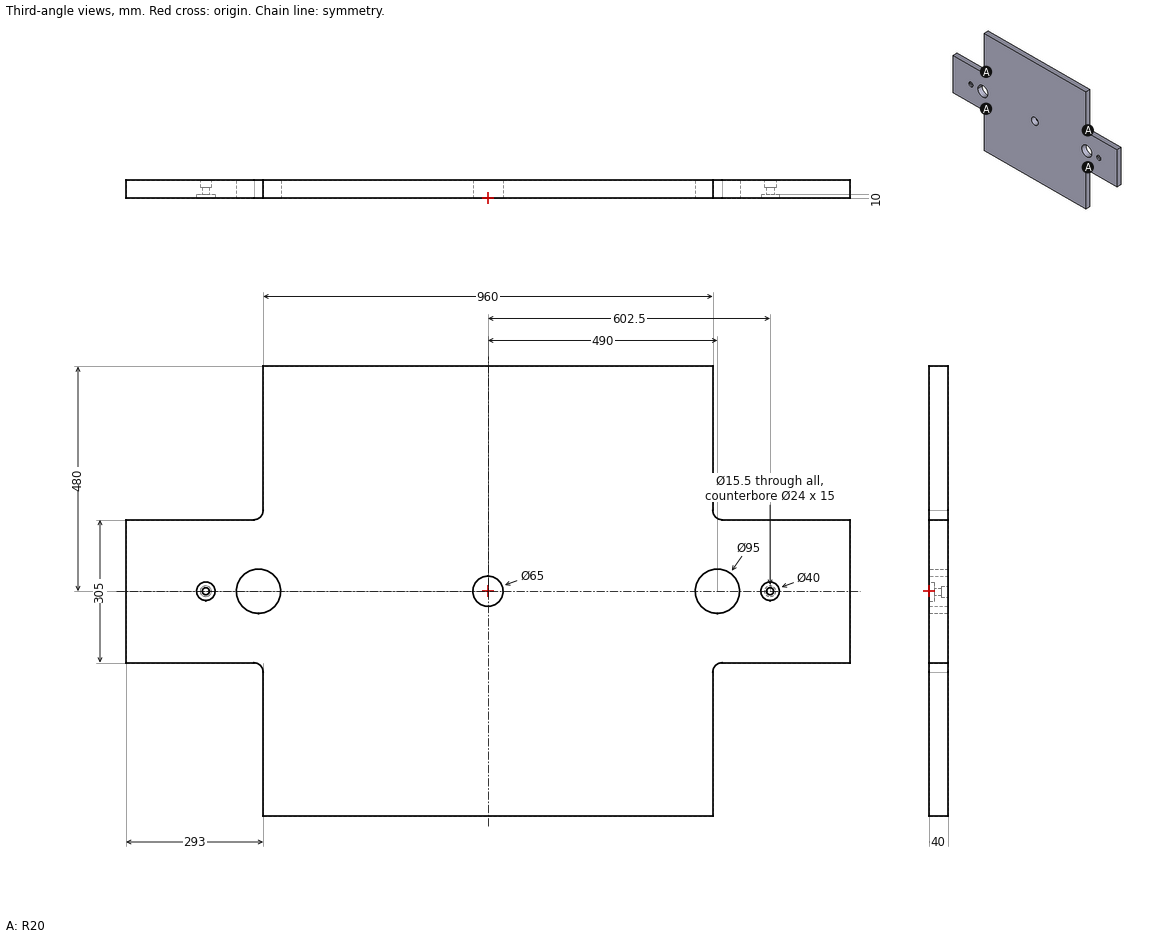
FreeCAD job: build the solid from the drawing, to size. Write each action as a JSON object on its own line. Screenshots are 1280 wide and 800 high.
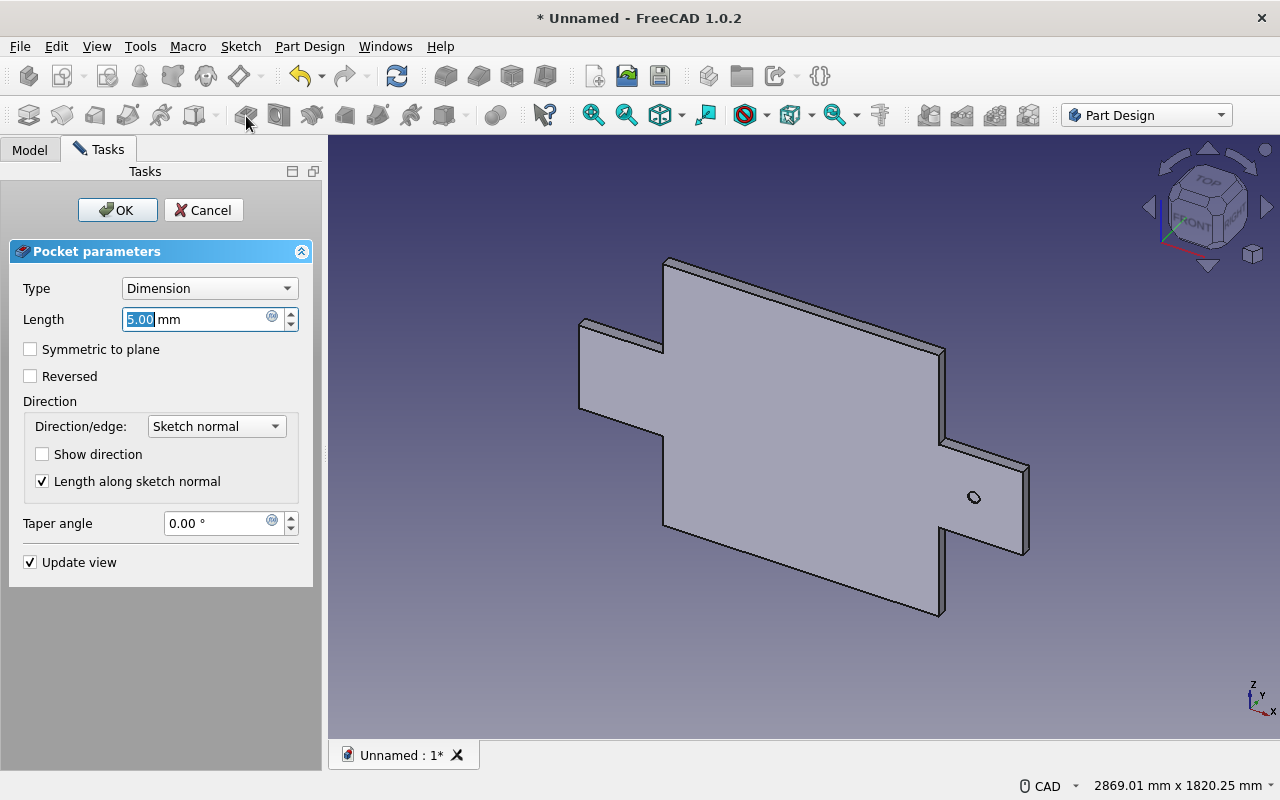
{"action": "type", "text": "10"}
{"action": "key", "text": "Tab"}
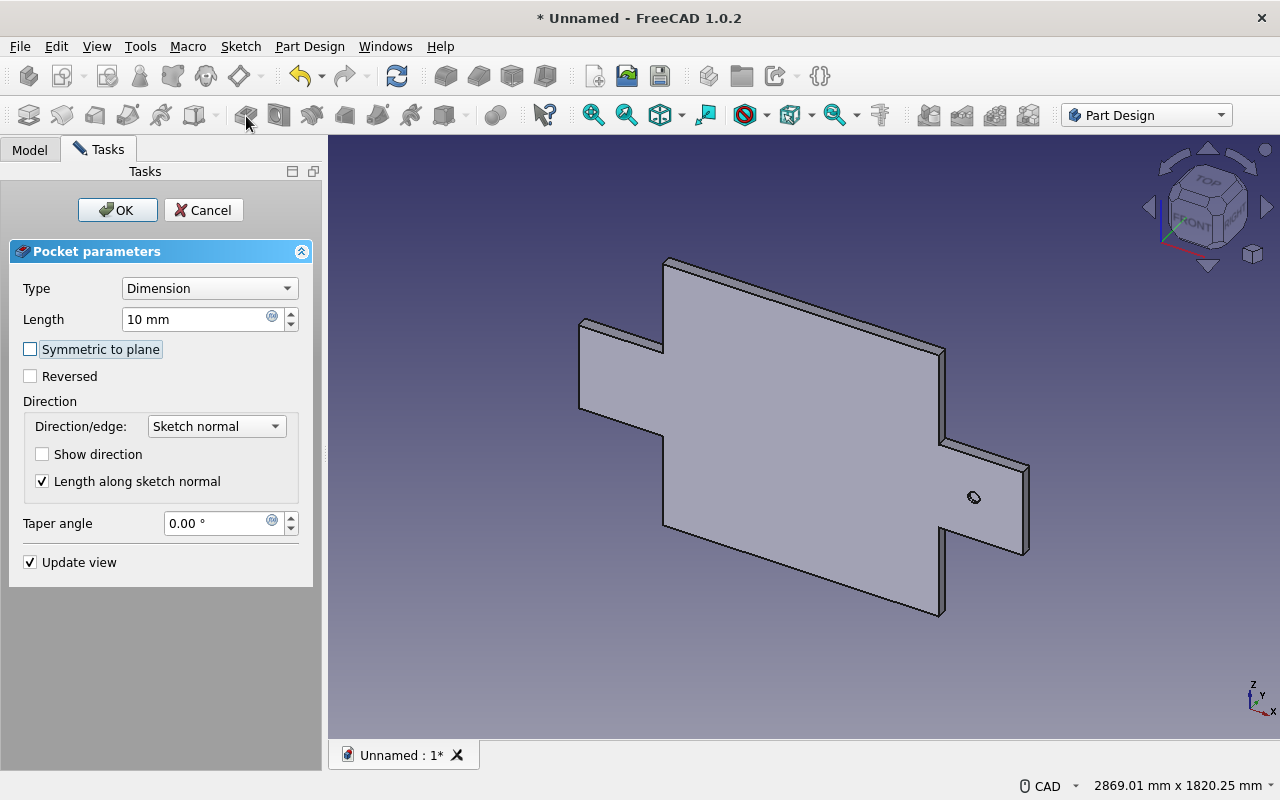
{"action": "left_click", "coordinate": [118, 210]}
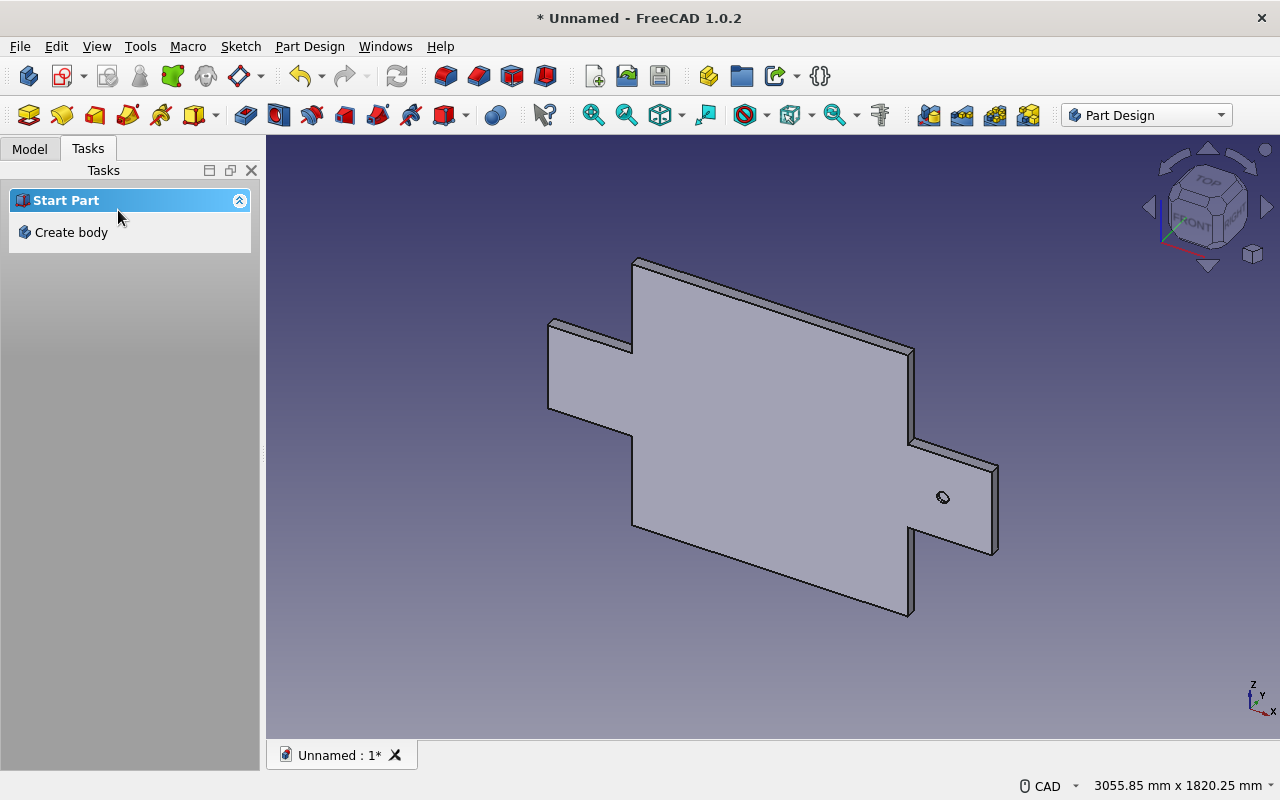
{"action": "key", "text": "4"}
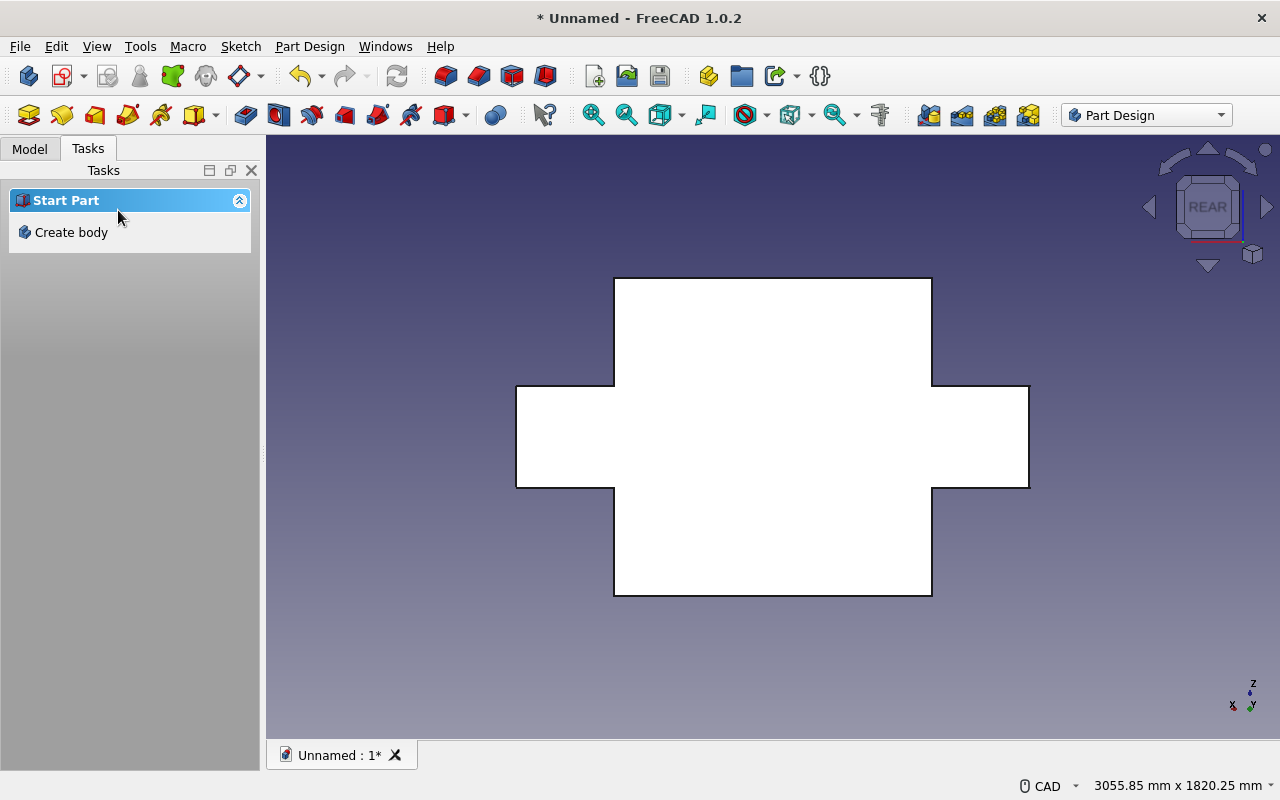
{"action": "left_click", "coordinate": [773, 436]}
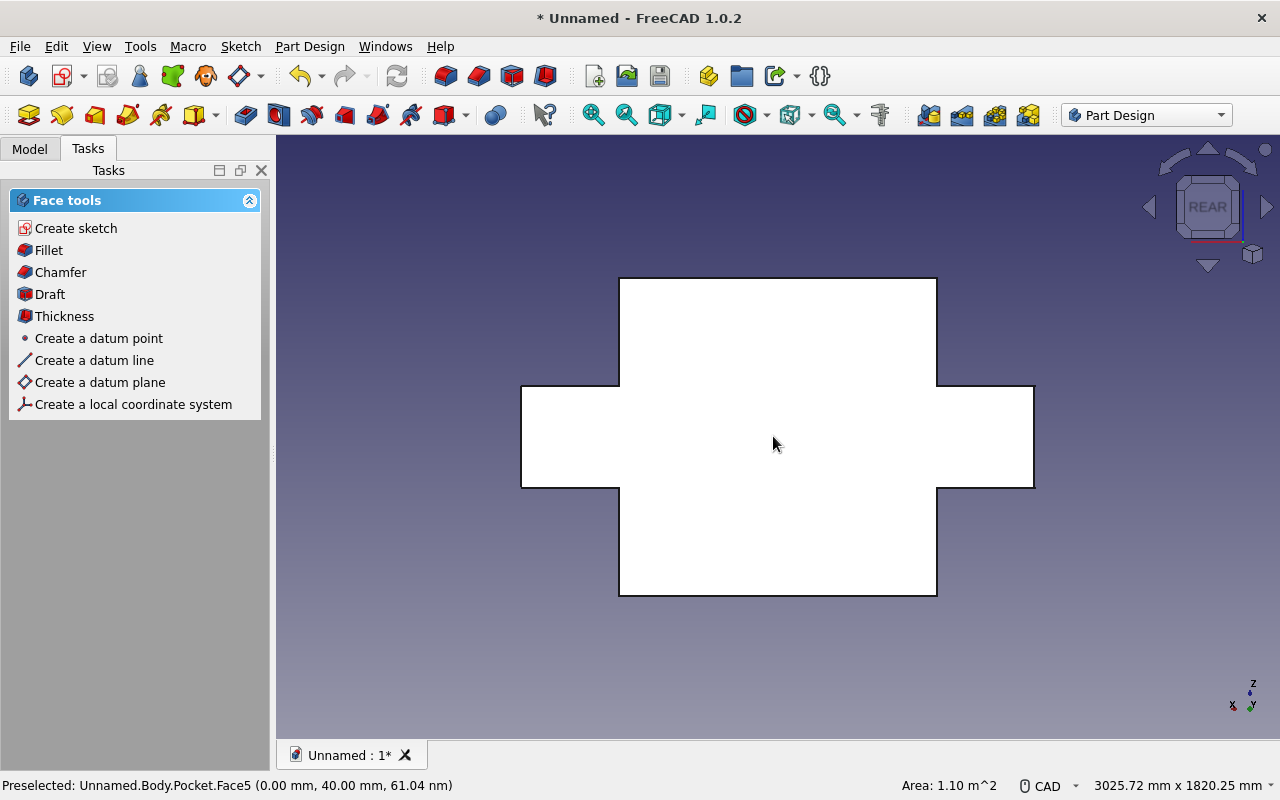
{"action": "left_click", "coordinate": [62, 76]}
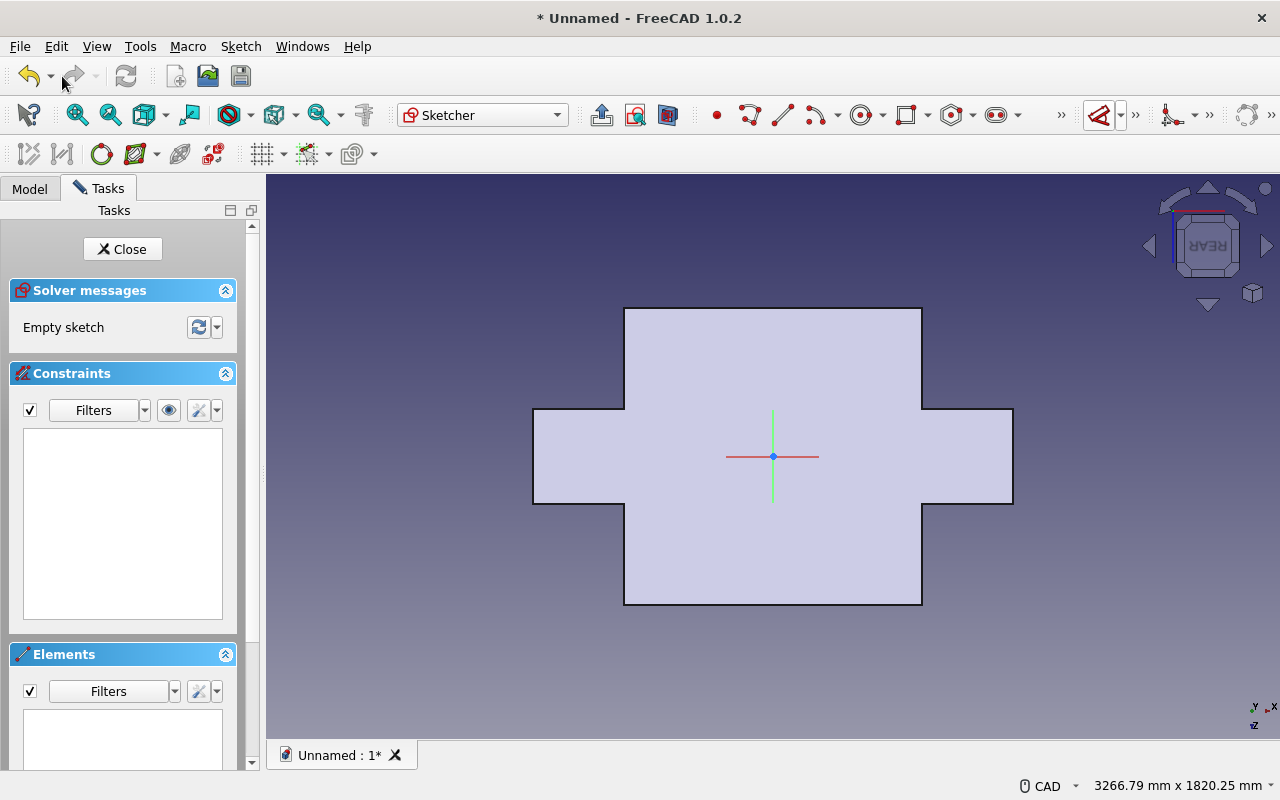
{"action": "scroll", "coordinate": [973, 456], "scroll_direction": "up", "scroll_amount": 15}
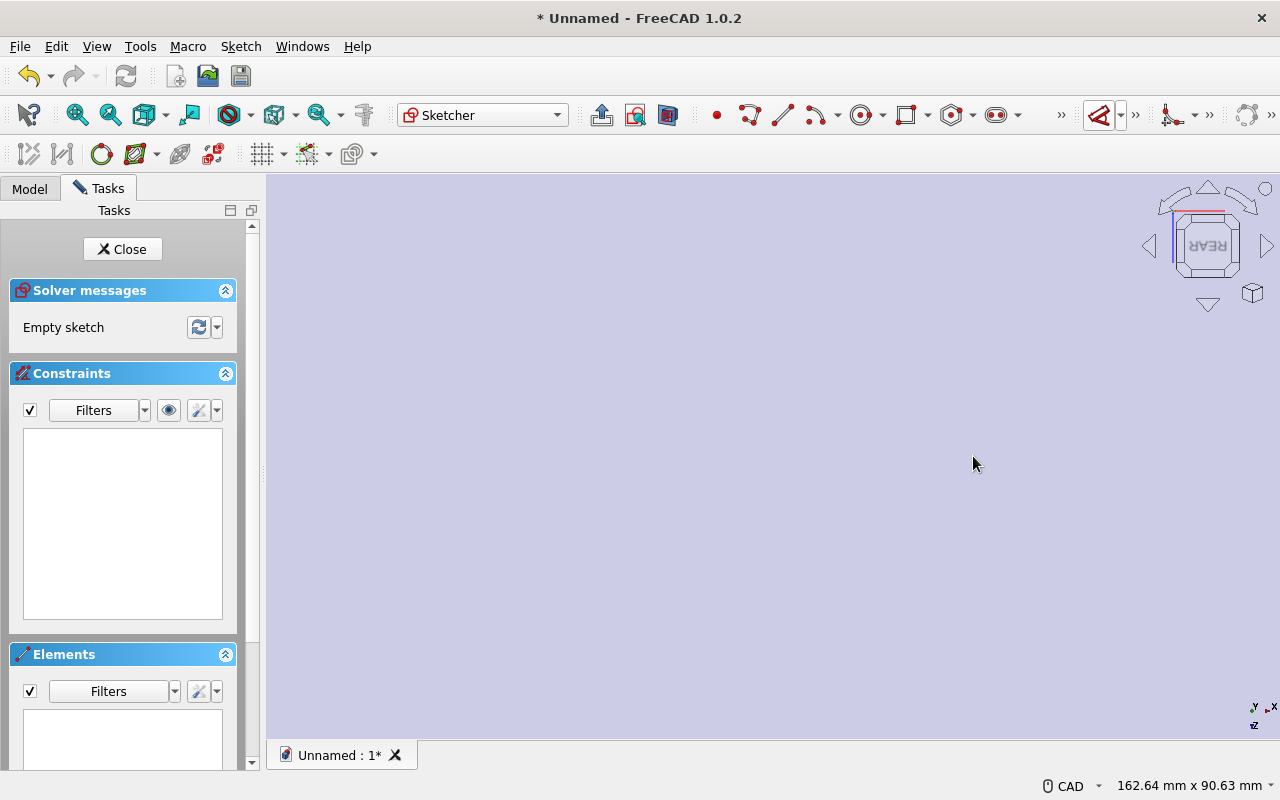
{"action": "scroll", "coordinate": [697, 456], "scroll_direction": "up", "scroll_amount": 7}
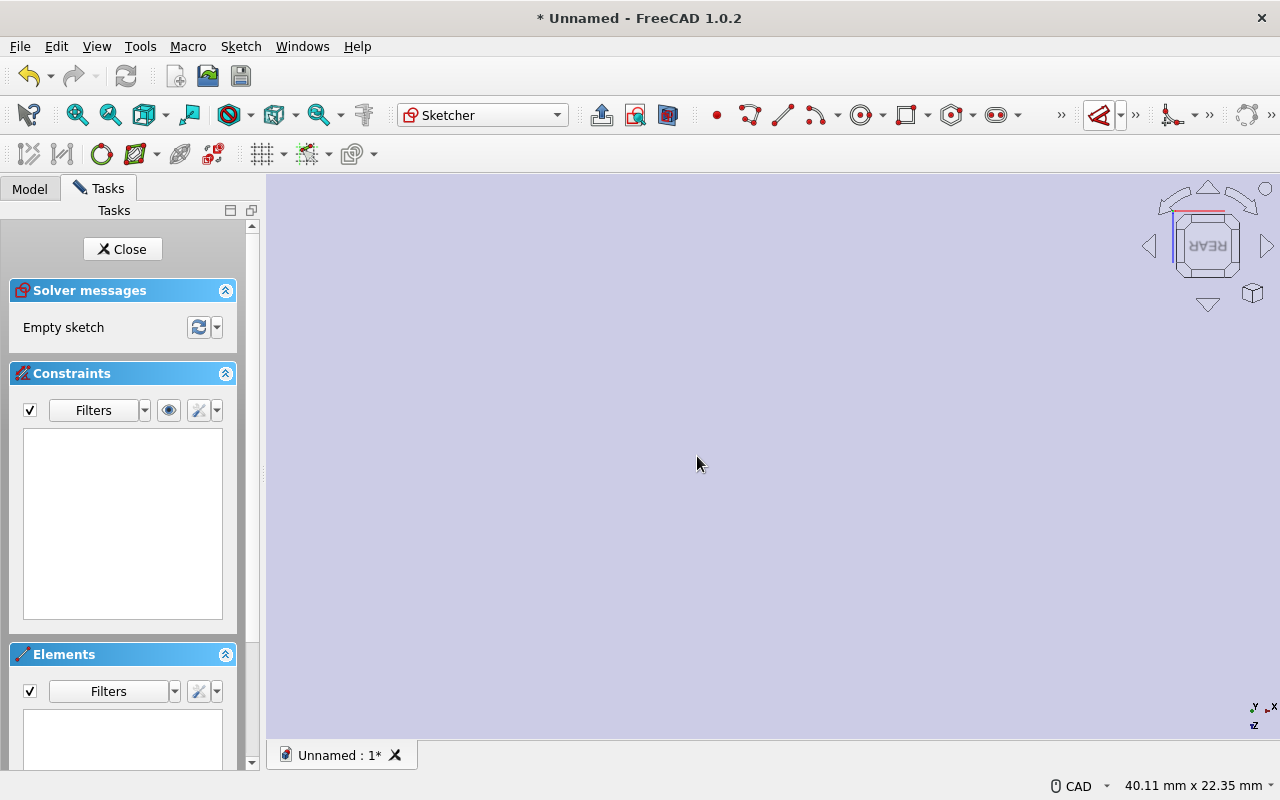
{"action": "key", "text": "g c"}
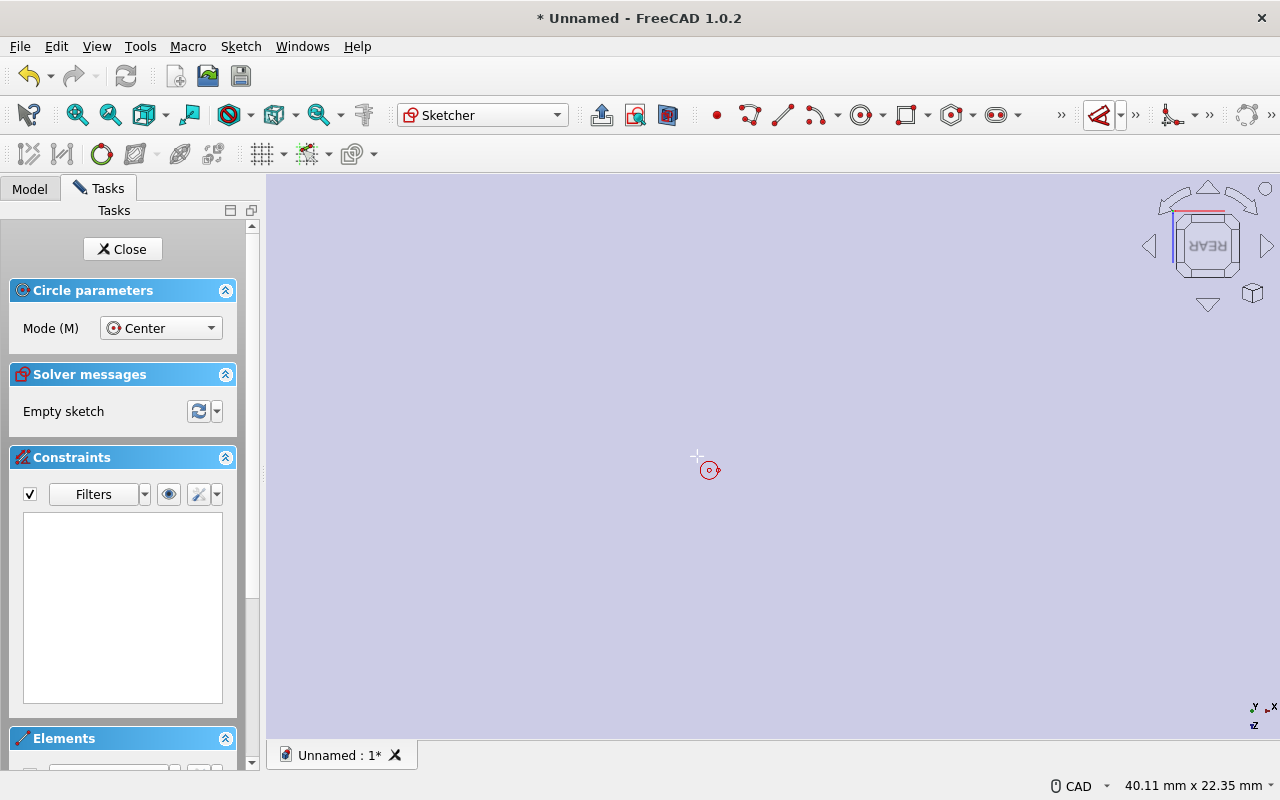
{"action": "left_click", "coordinate": [703, 456]}
{"action": "mouse_move", "coordinate": [842, 318]}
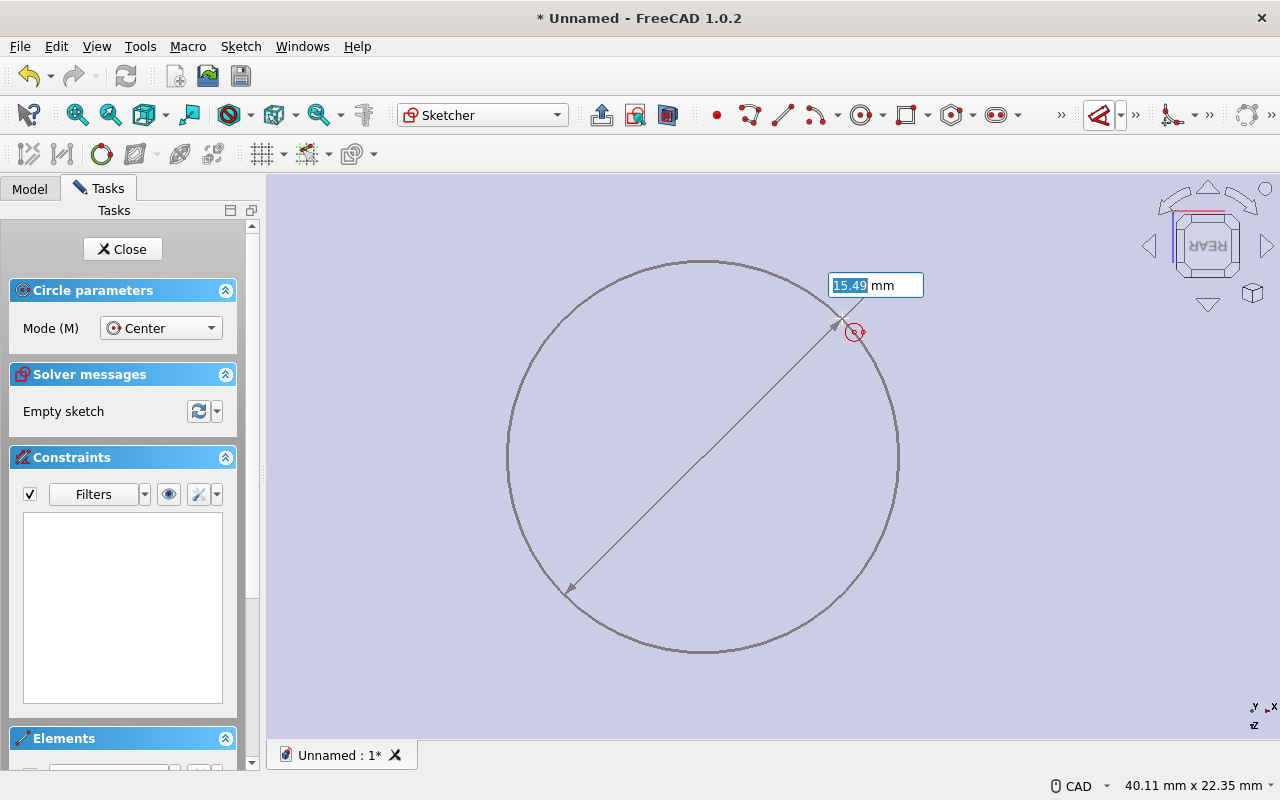
{"action": "type", "text": "15.5"}
{"action": "key", "text": "Return"}
{"action": "key", "text": "Escape"}